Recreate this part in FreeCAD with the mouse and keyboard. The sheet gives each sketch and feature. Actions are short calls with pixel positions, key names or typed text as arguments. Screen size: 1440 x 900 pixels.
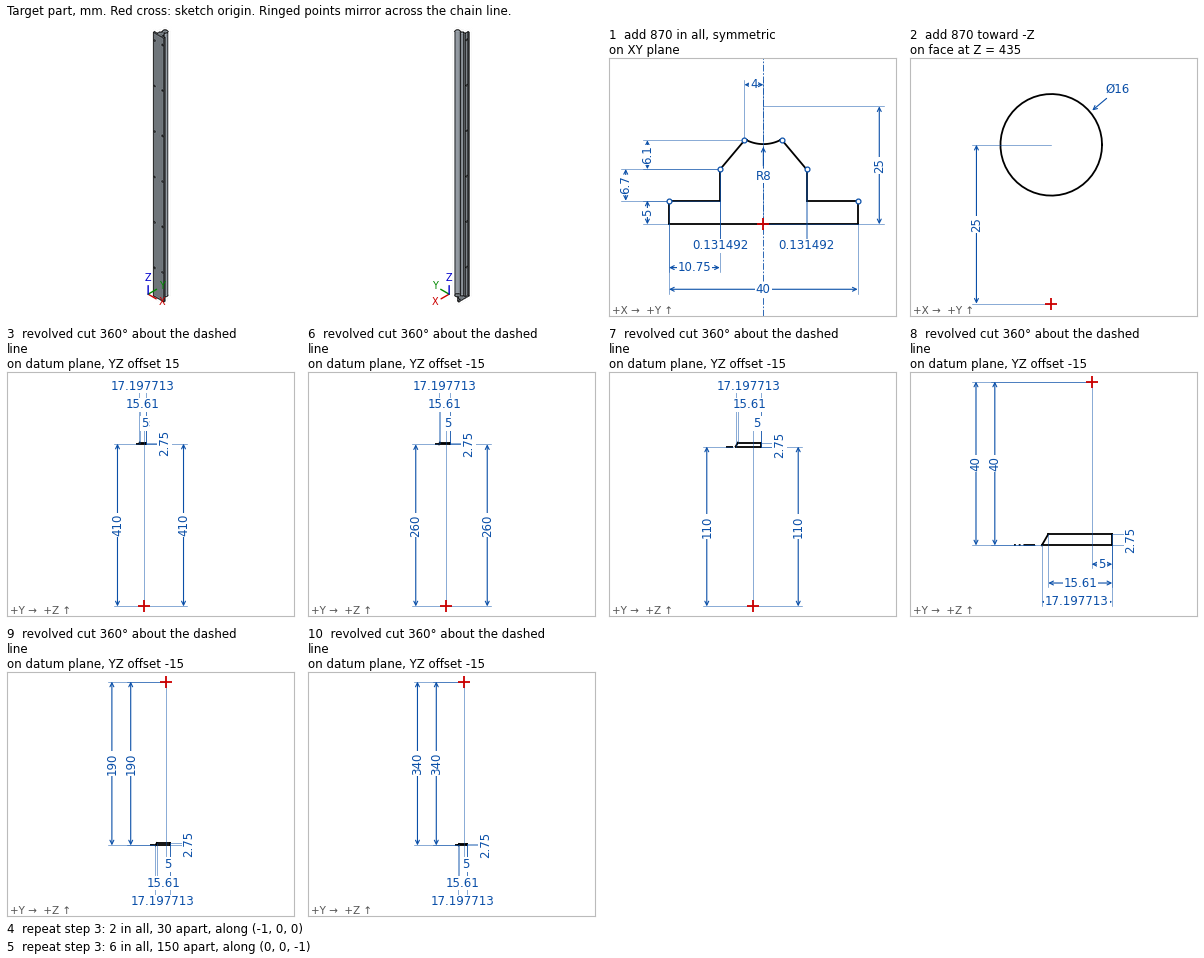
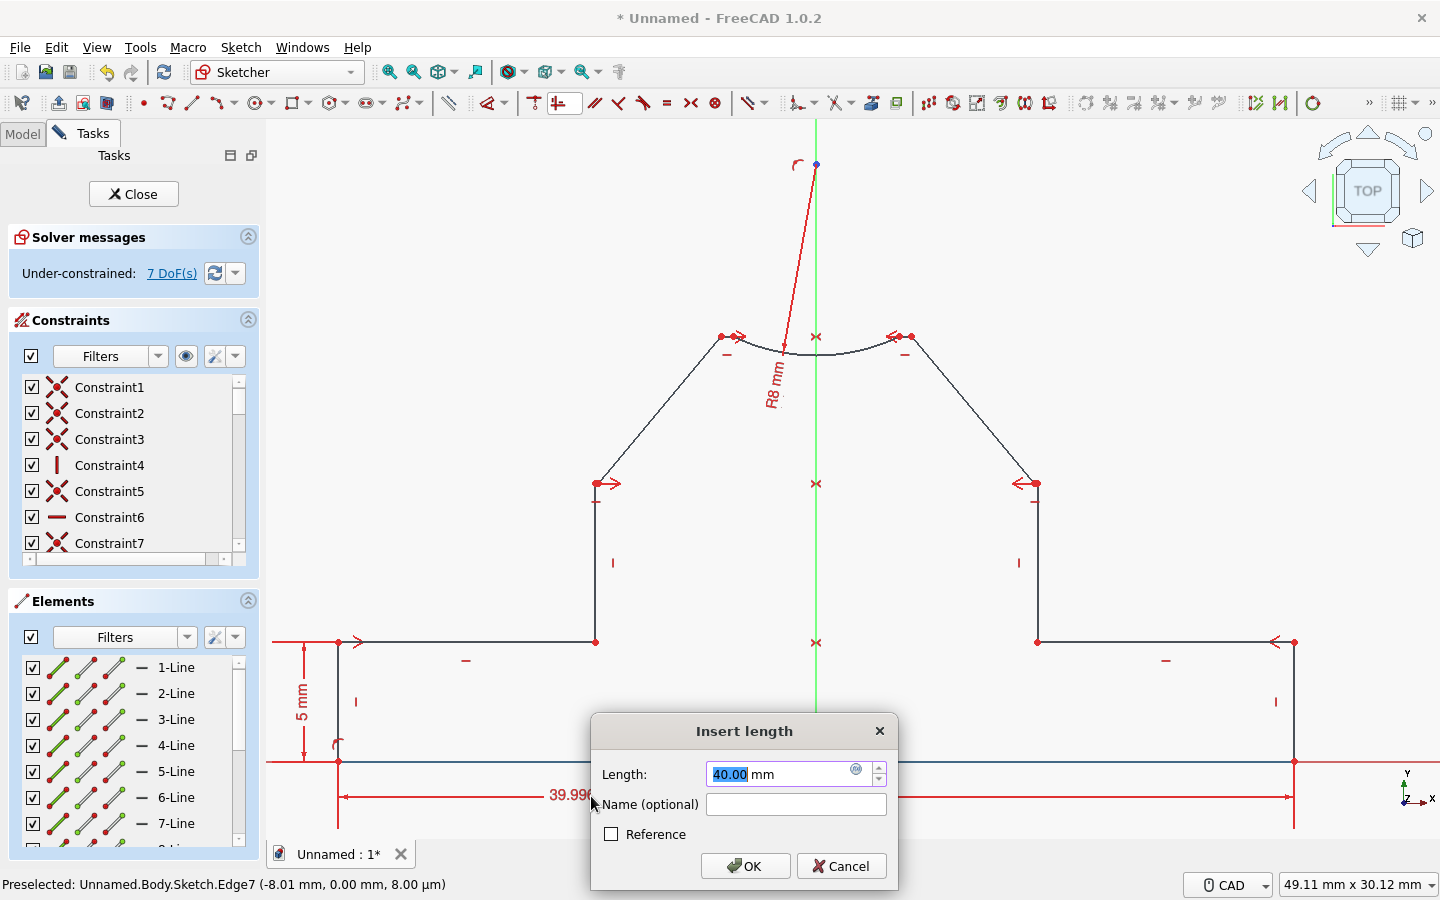
text(40)
key(Return)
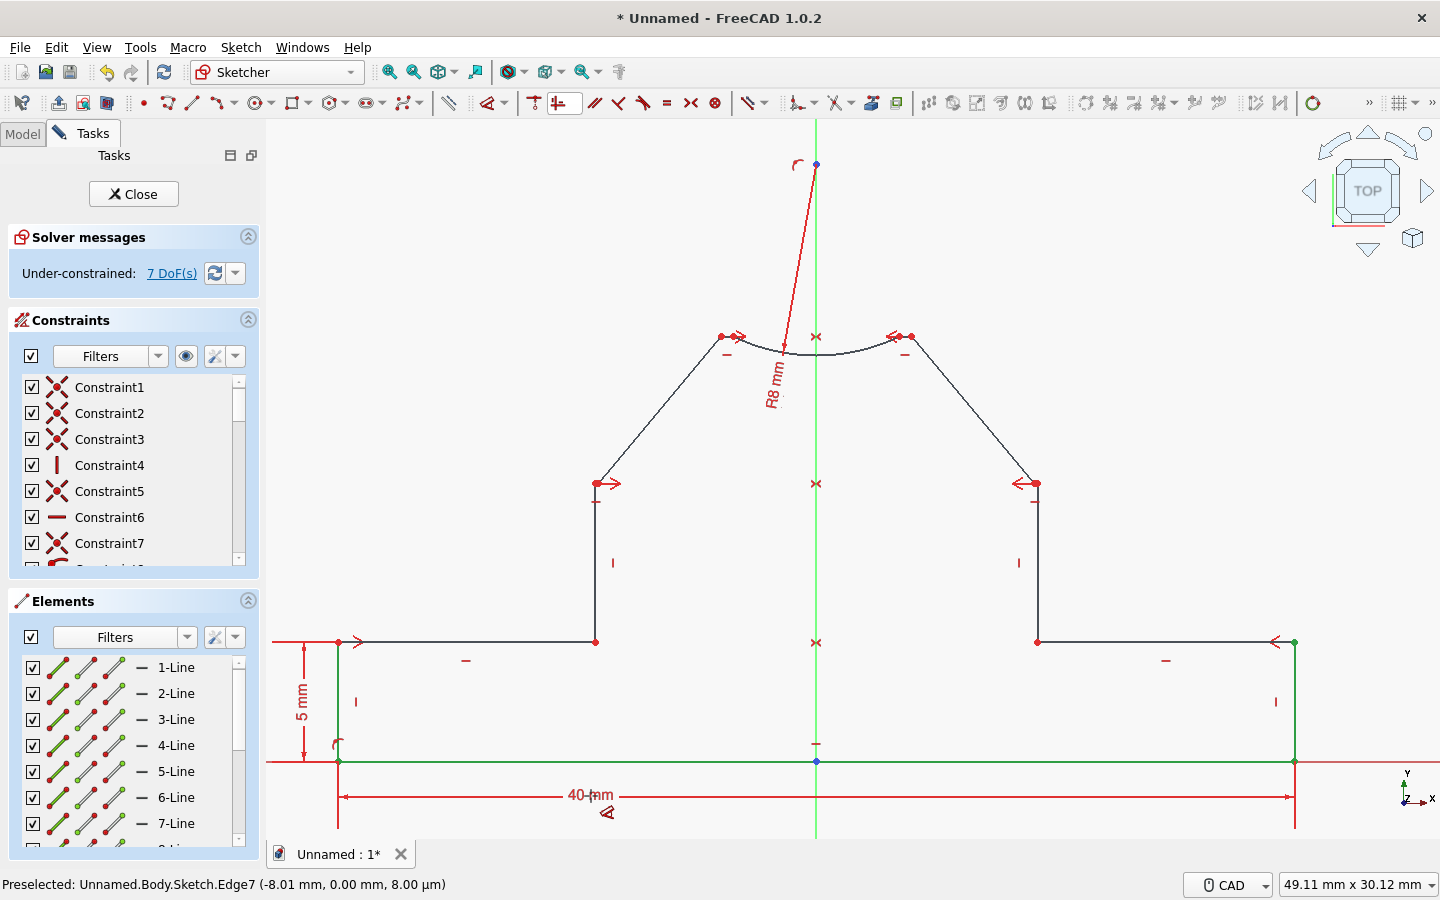
click(721, 337)
click(769, 796)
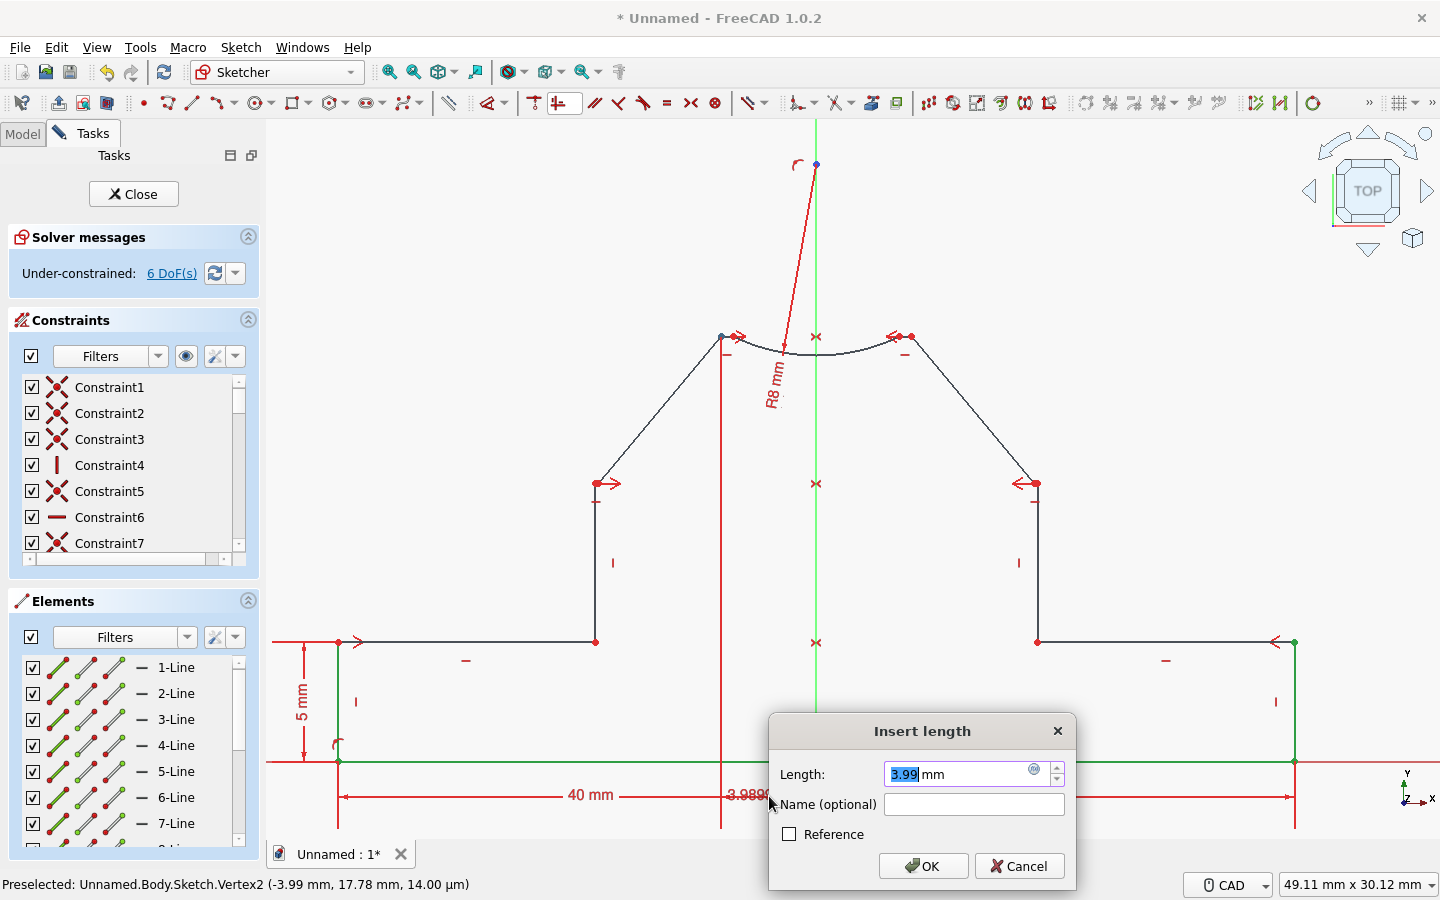
text(4)
key(Return)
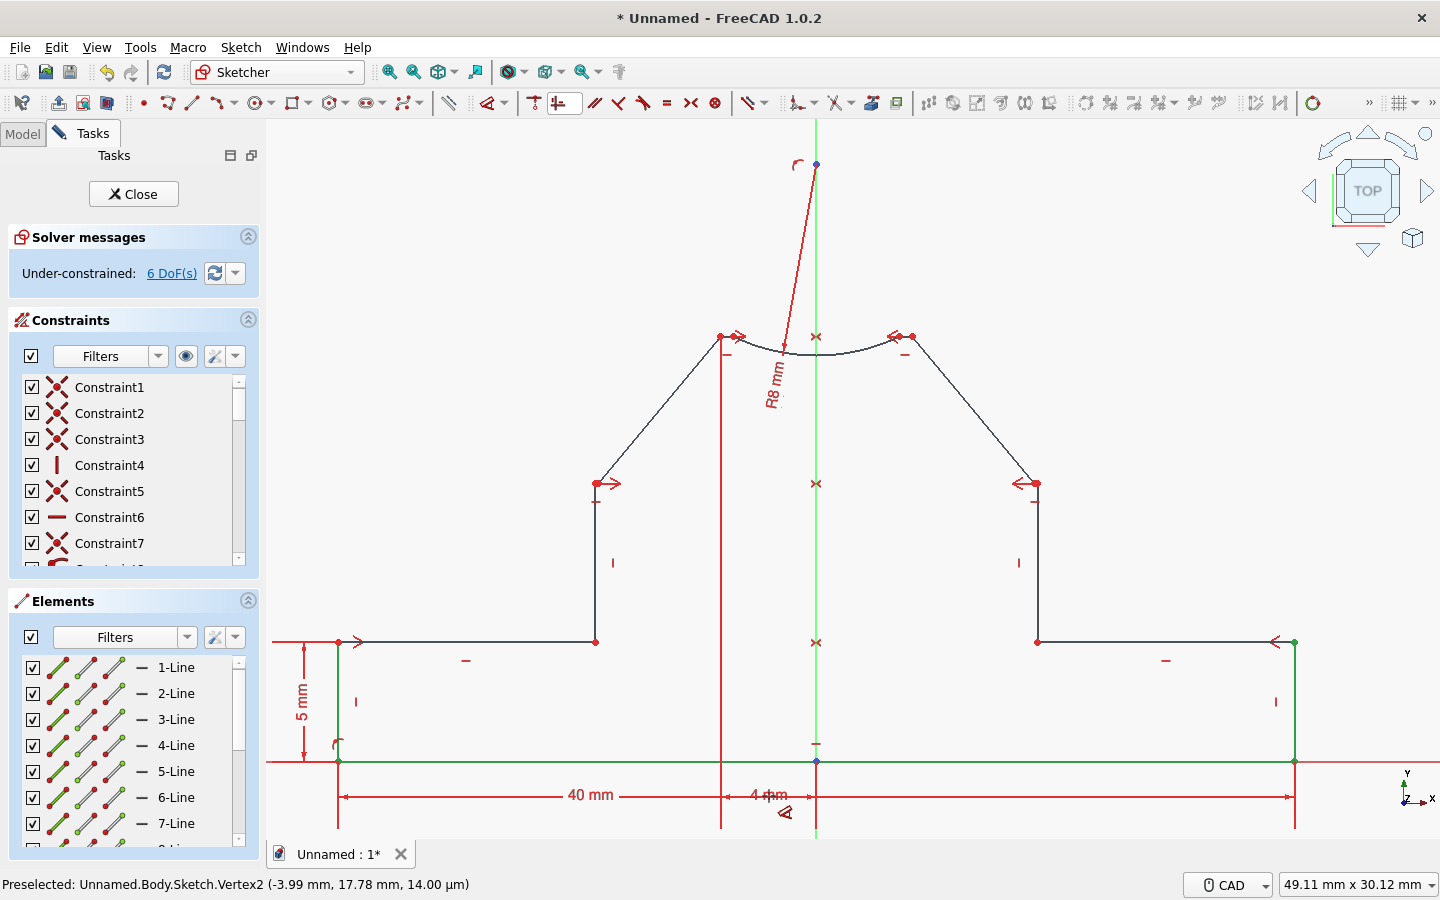
click(595, 531)
click(561, 563)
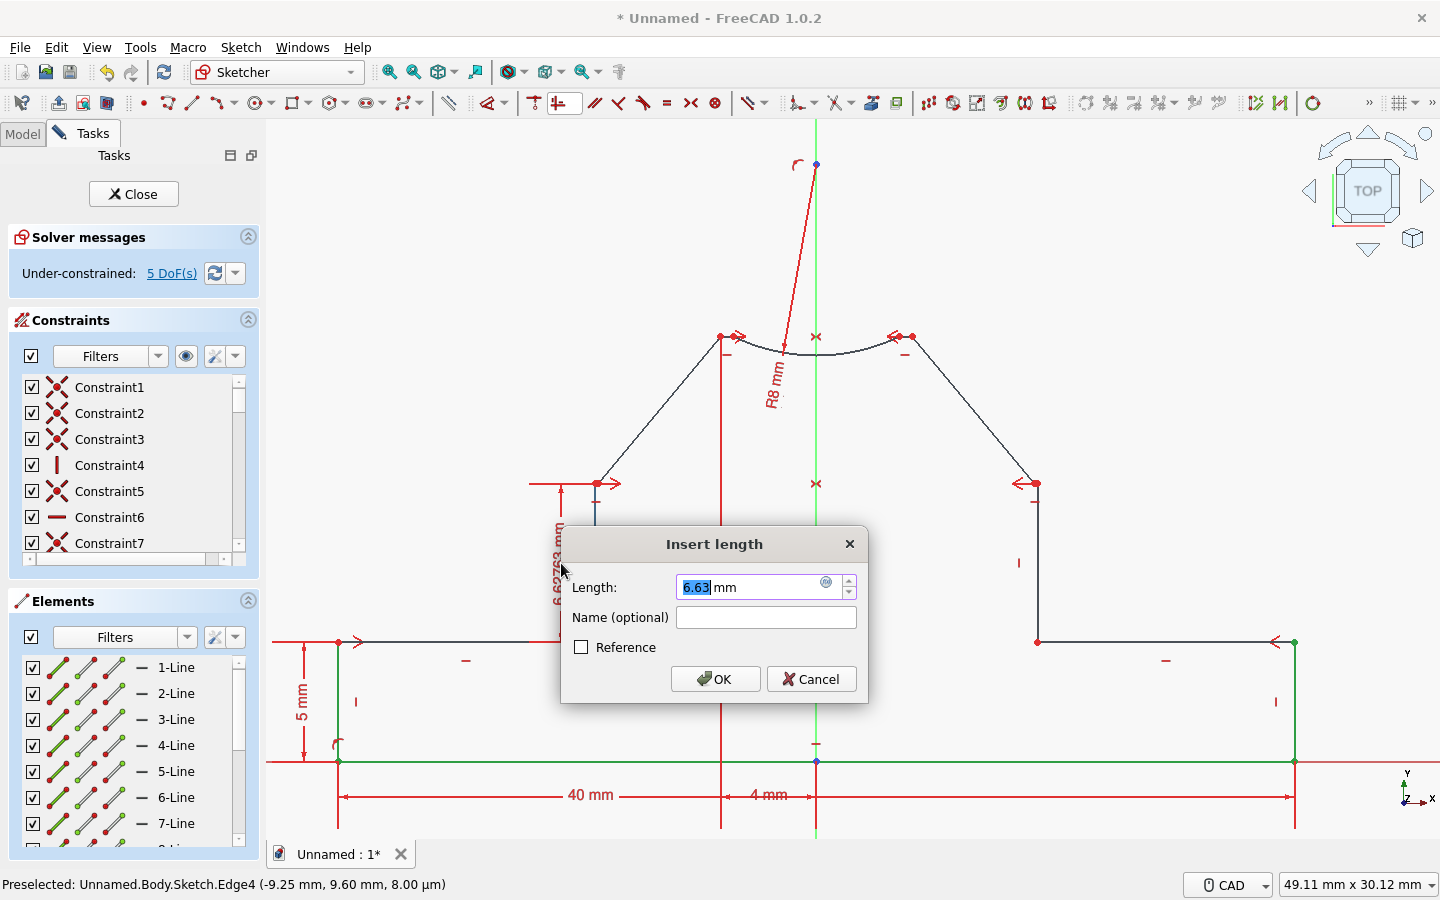
text(6.7)
key(Return)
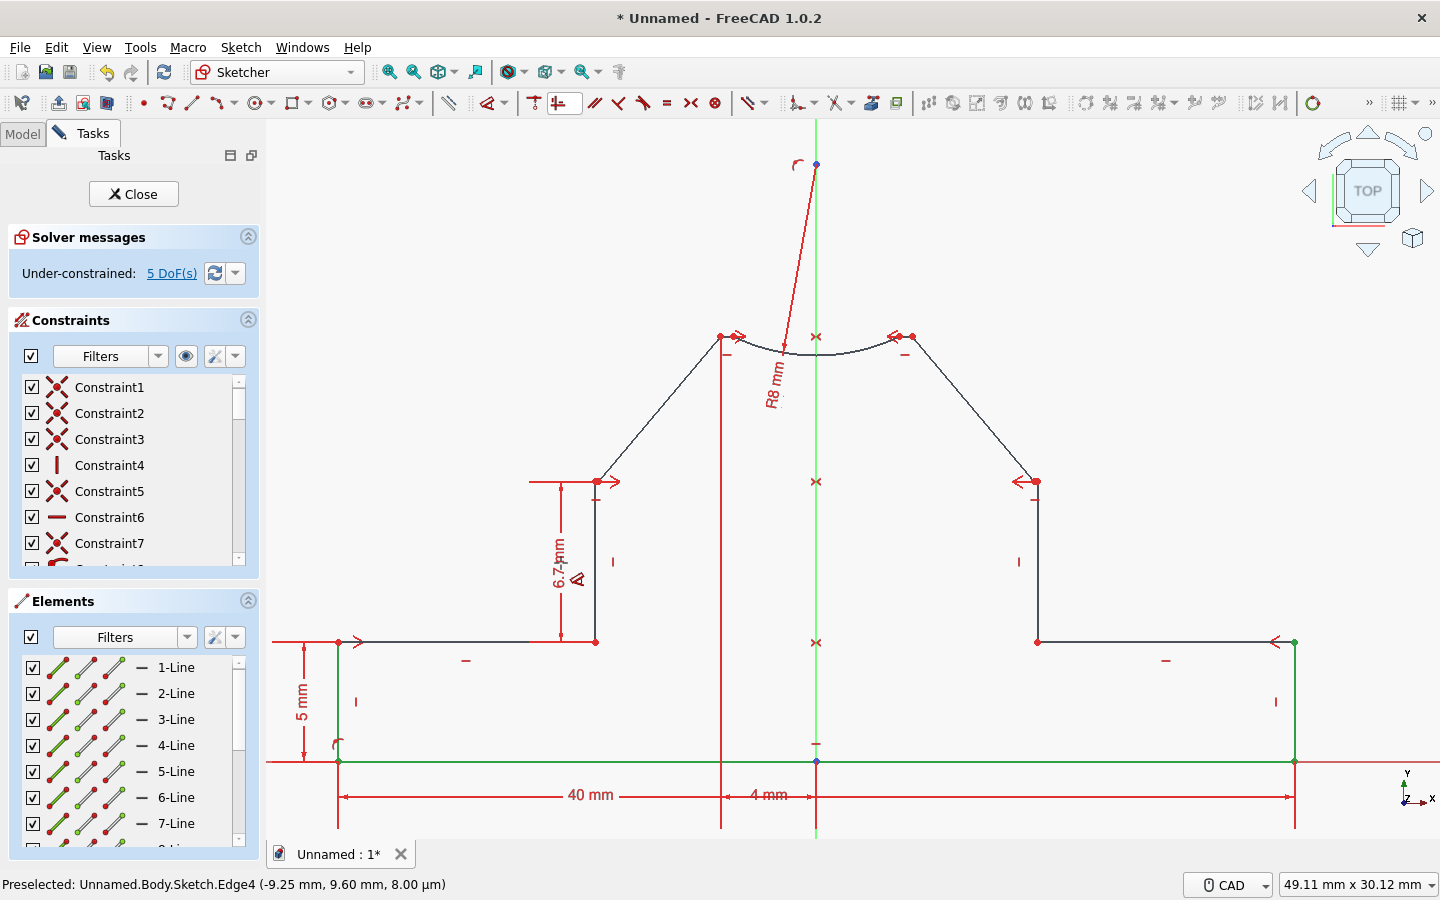
click(816, 164)
click(850, 463)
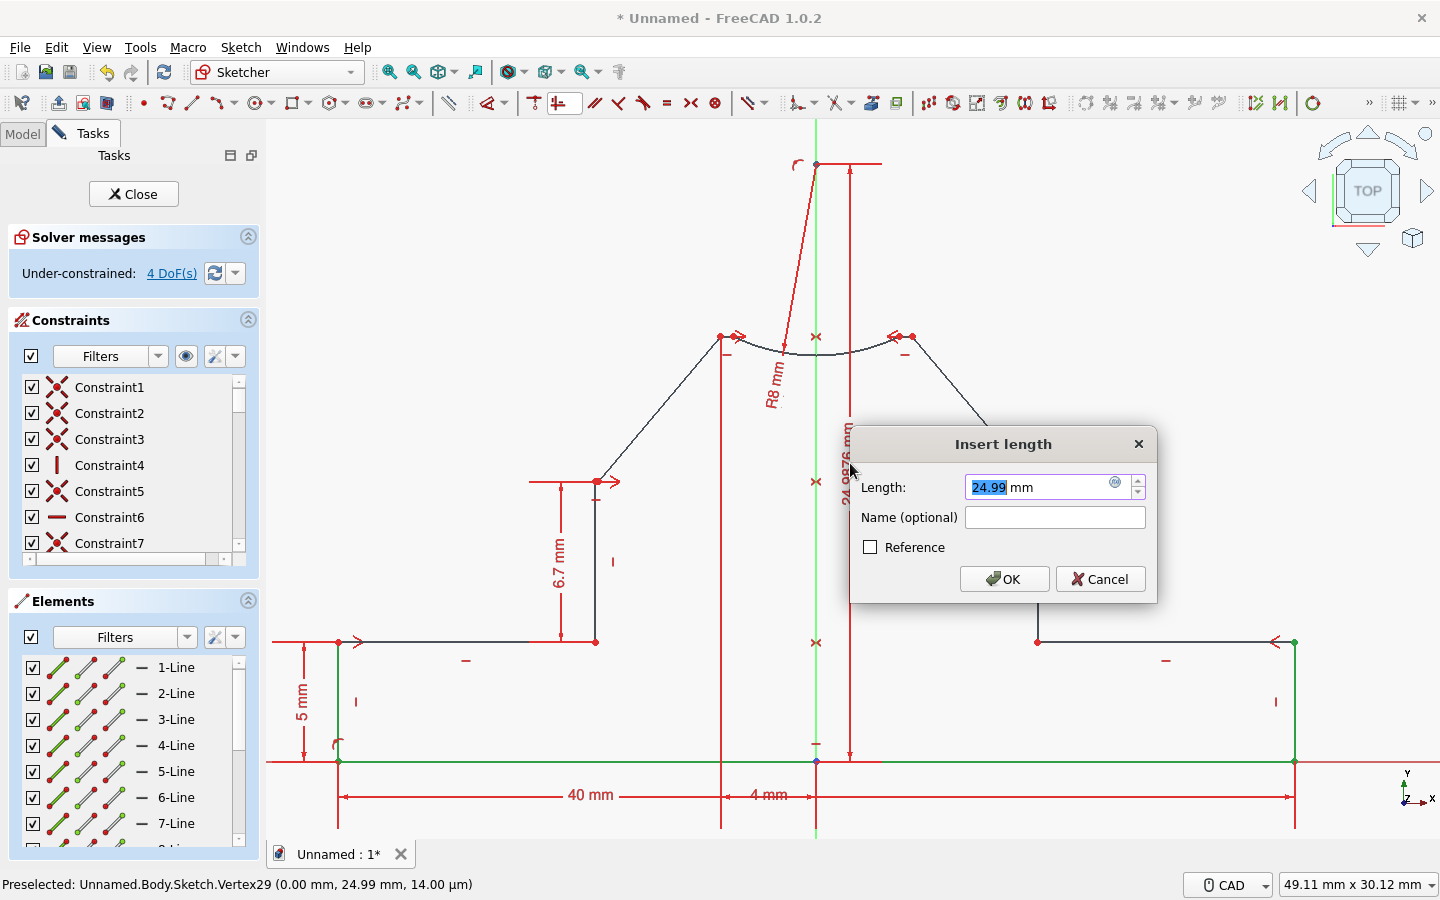
text(25)
key(Return)